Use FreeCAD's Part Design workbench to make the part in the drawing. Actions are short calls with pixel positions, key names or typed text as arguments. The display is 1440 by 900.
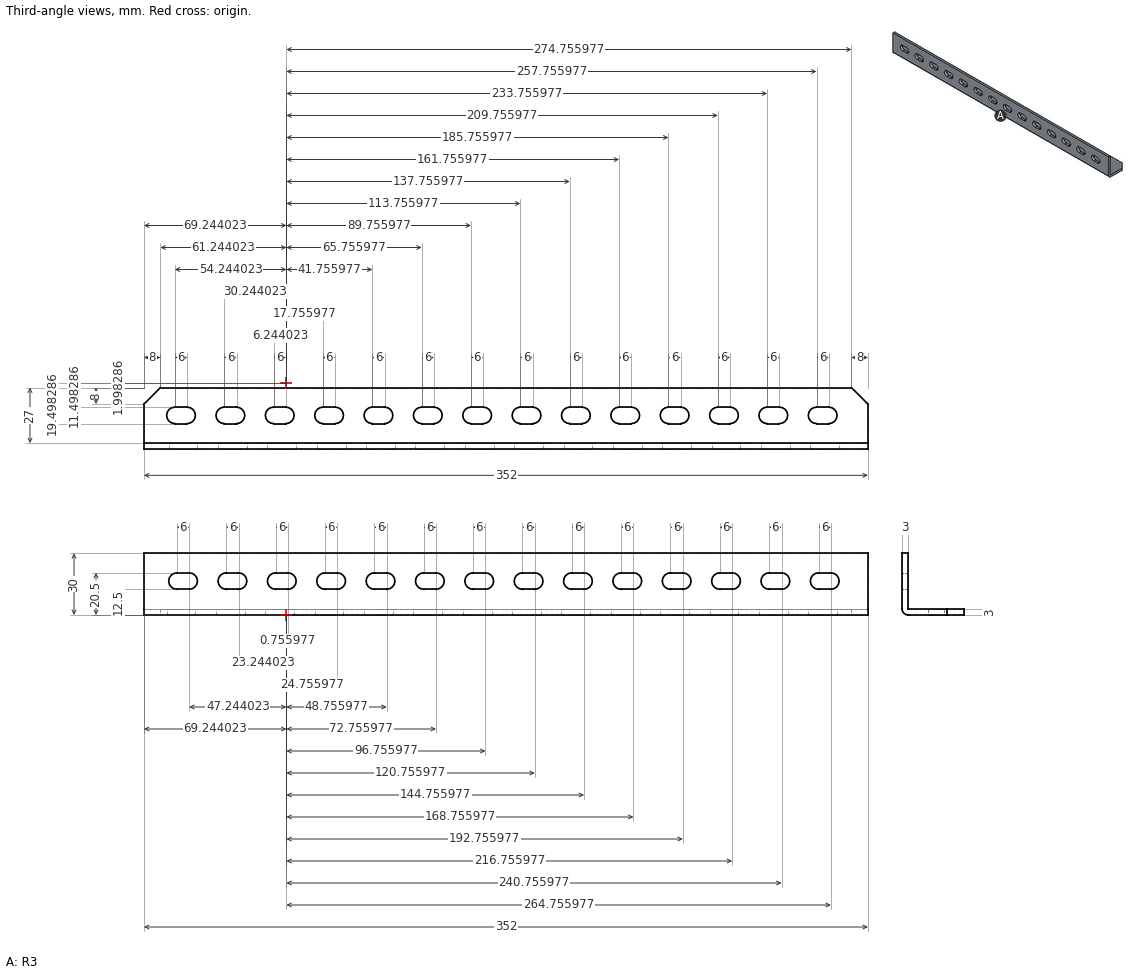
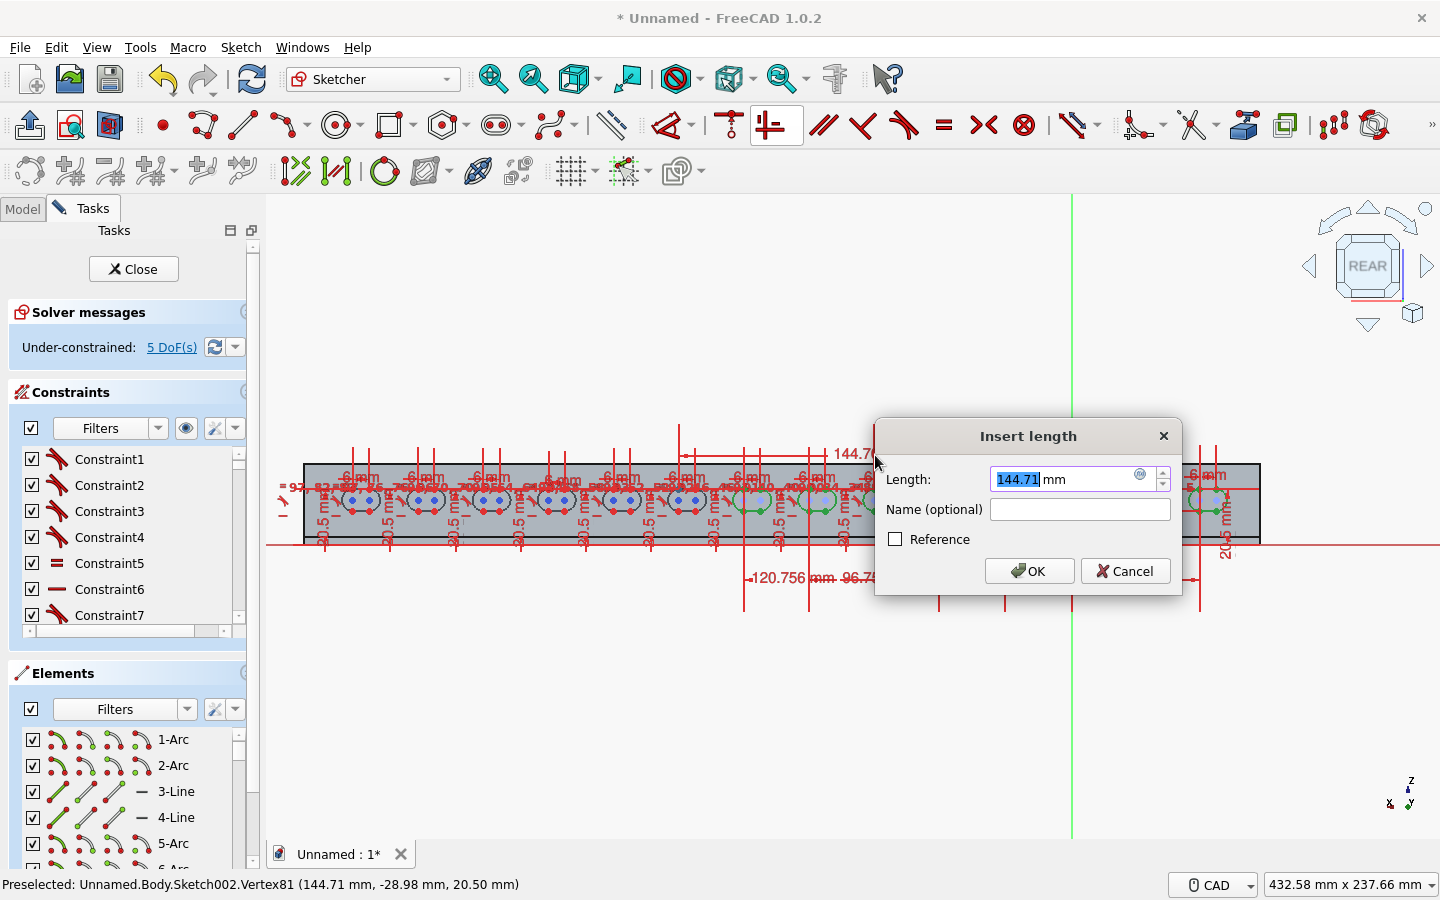
text(144.755977)
key(Return)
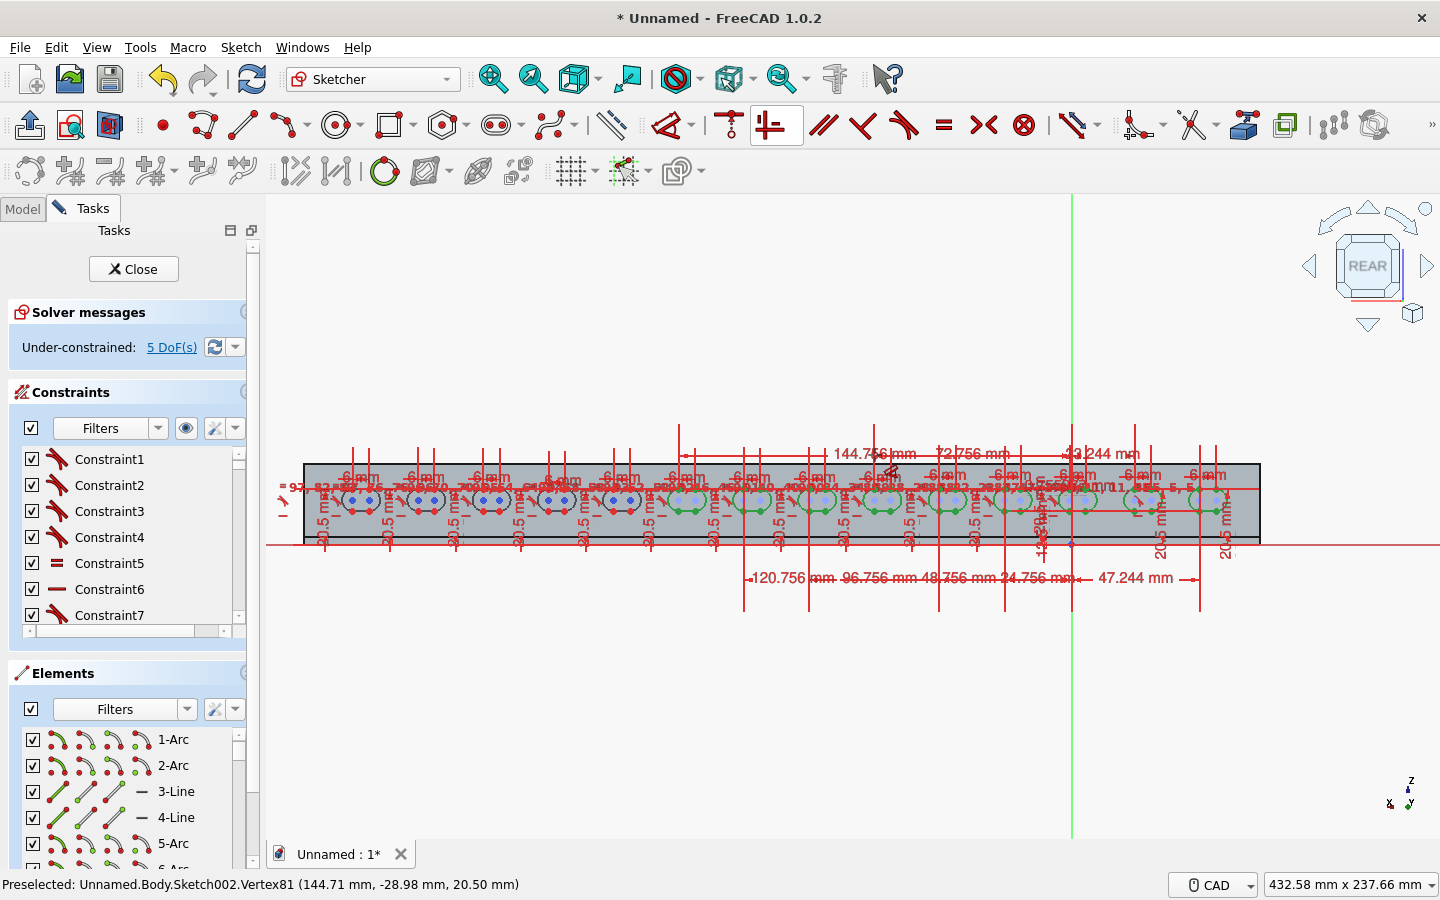
click(614, 489)
click(683, 579)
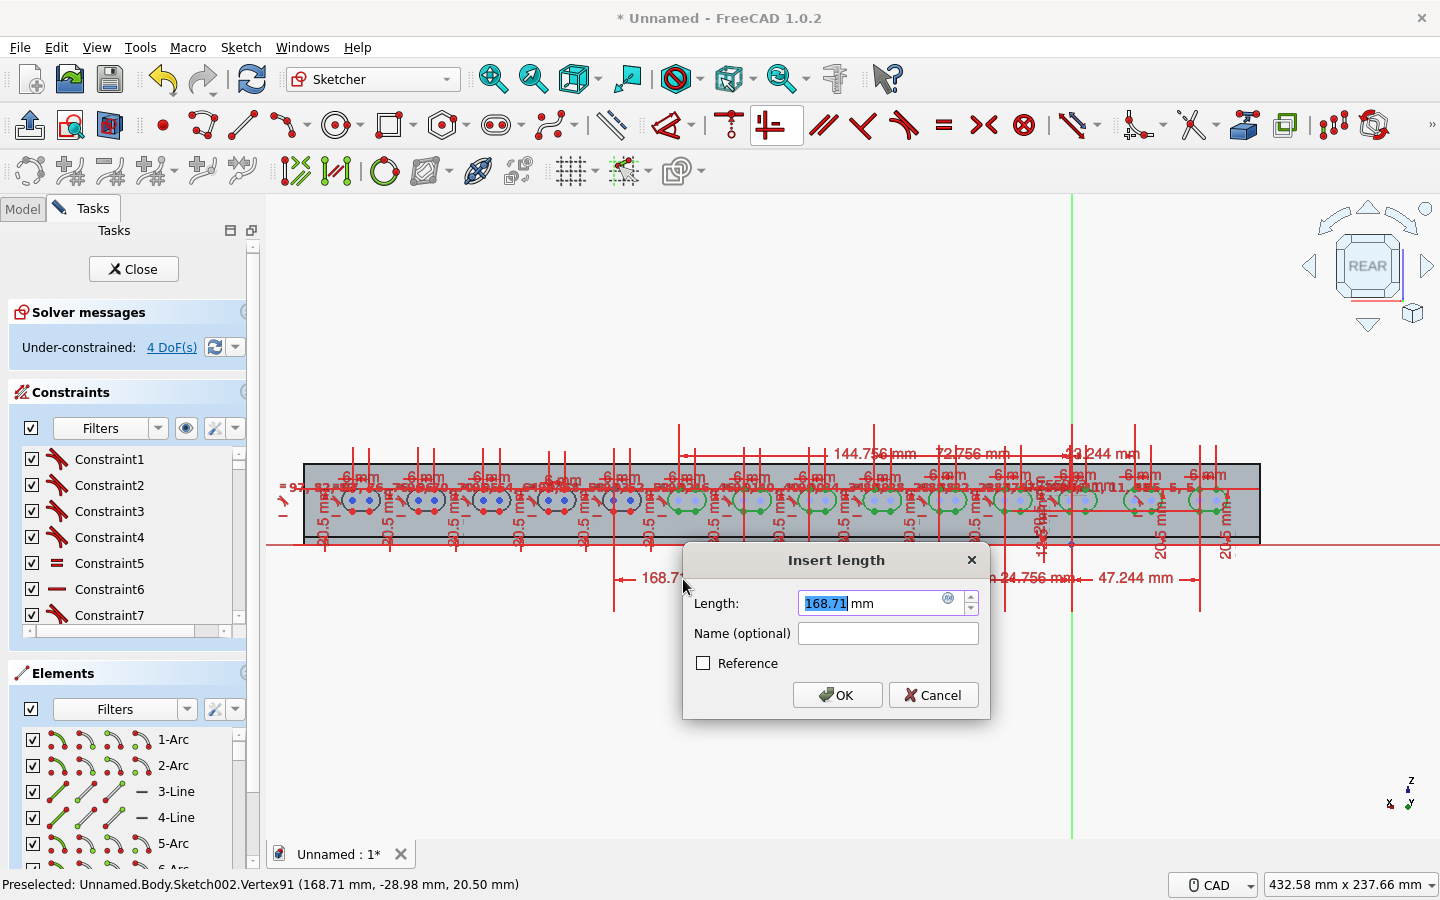
text(168.755977)
key(Return)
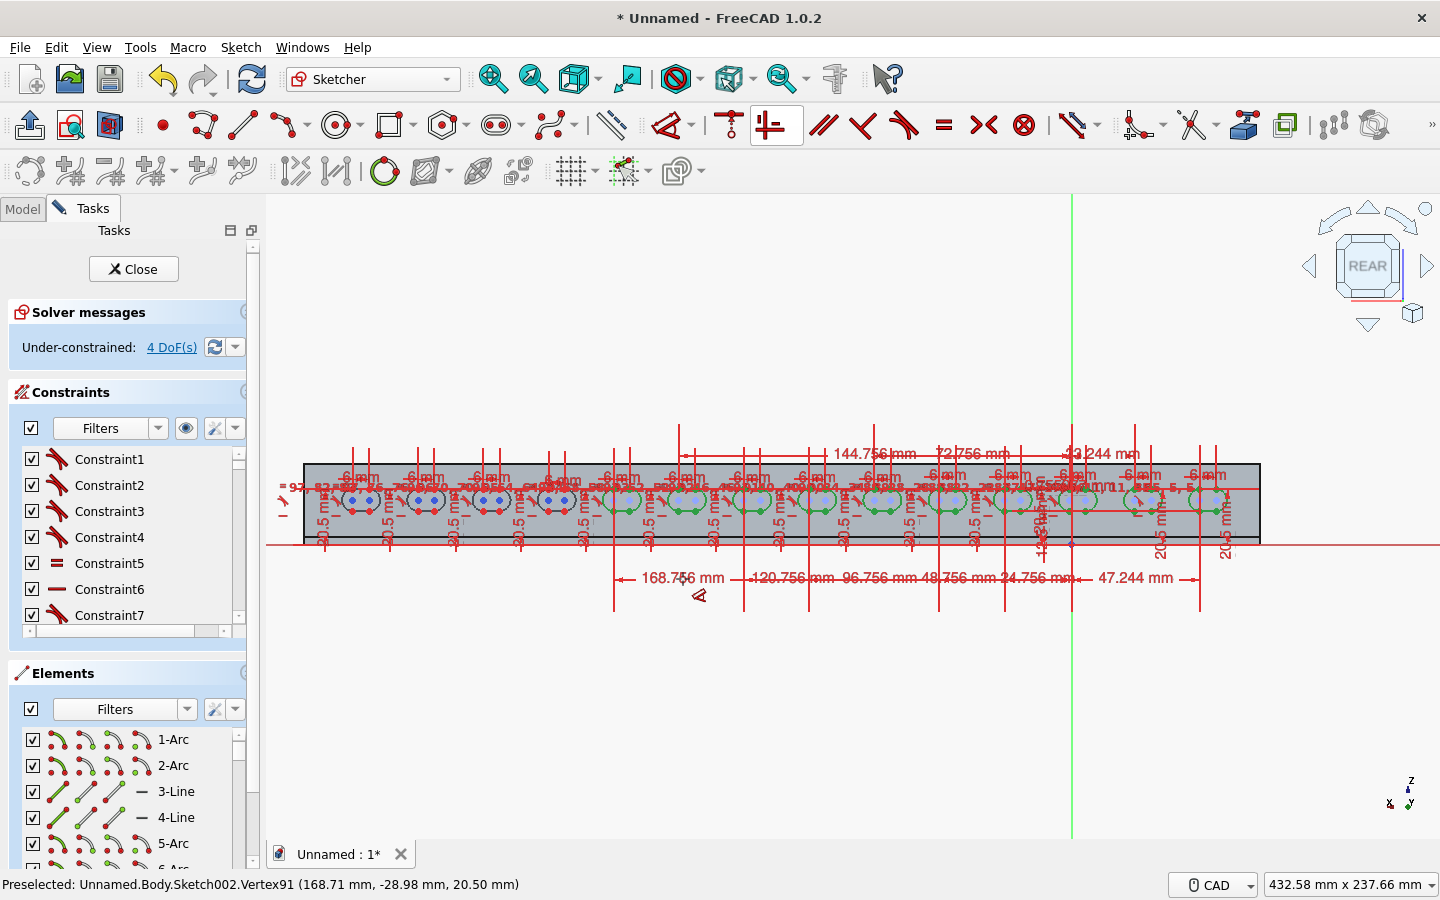
click(549, 489)
click(690, 455)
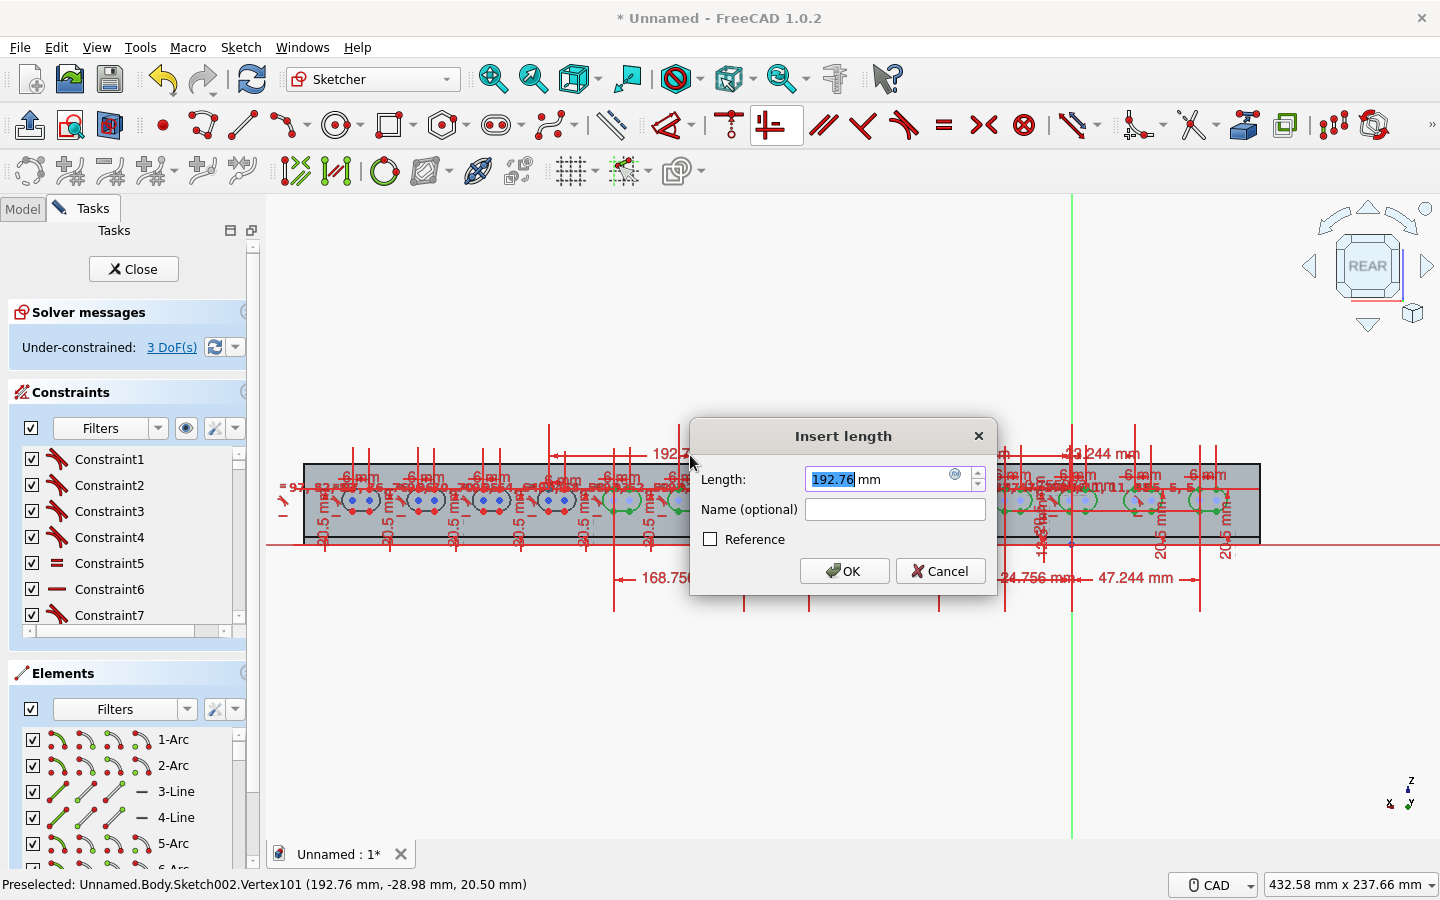
text(192.755977)
key(Return)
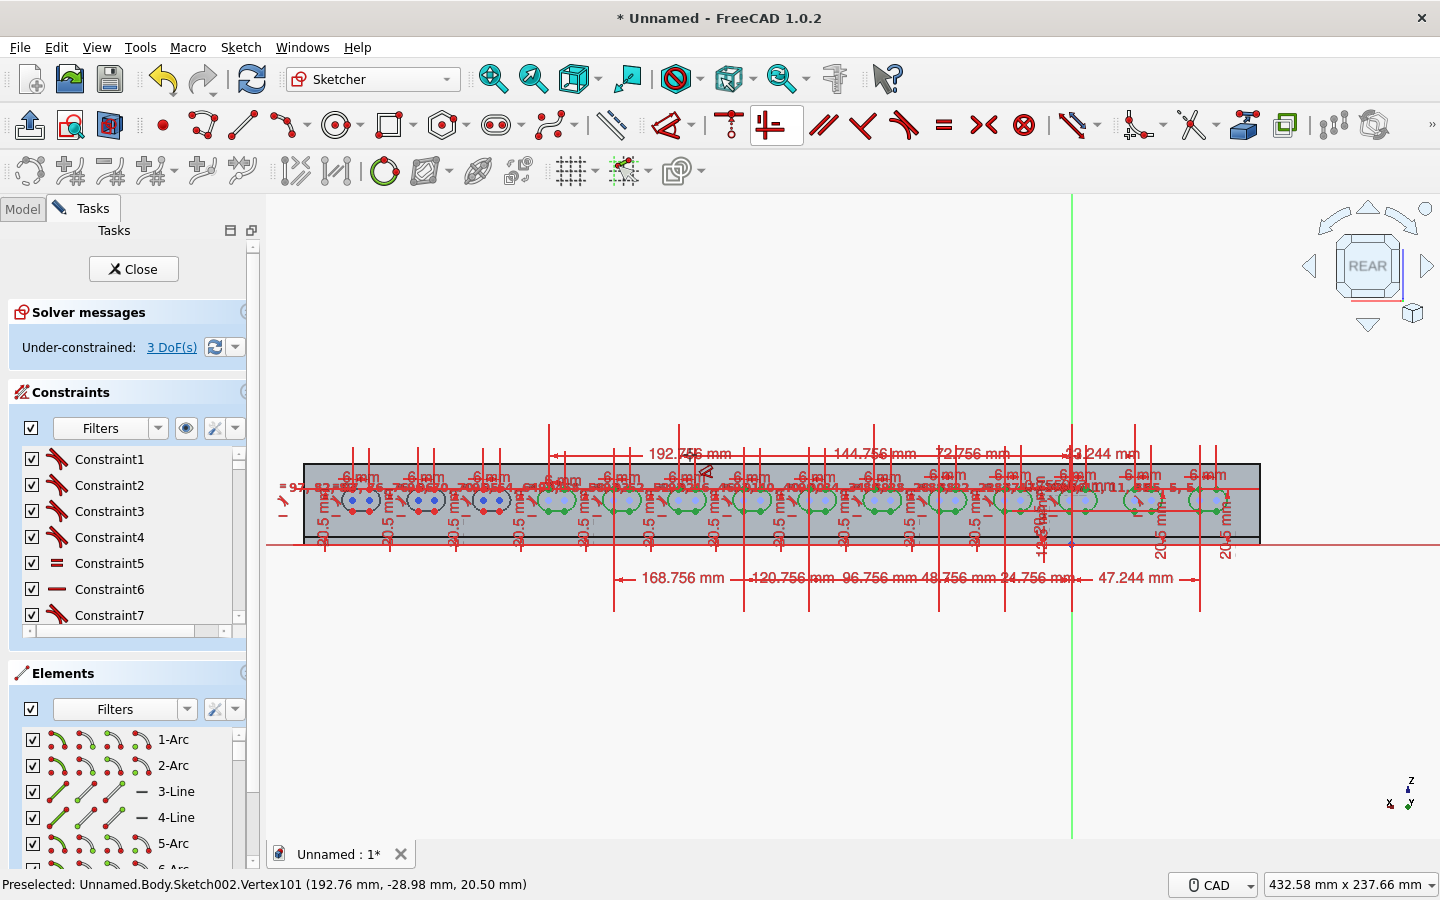
click(483, 489)
click(572, 579)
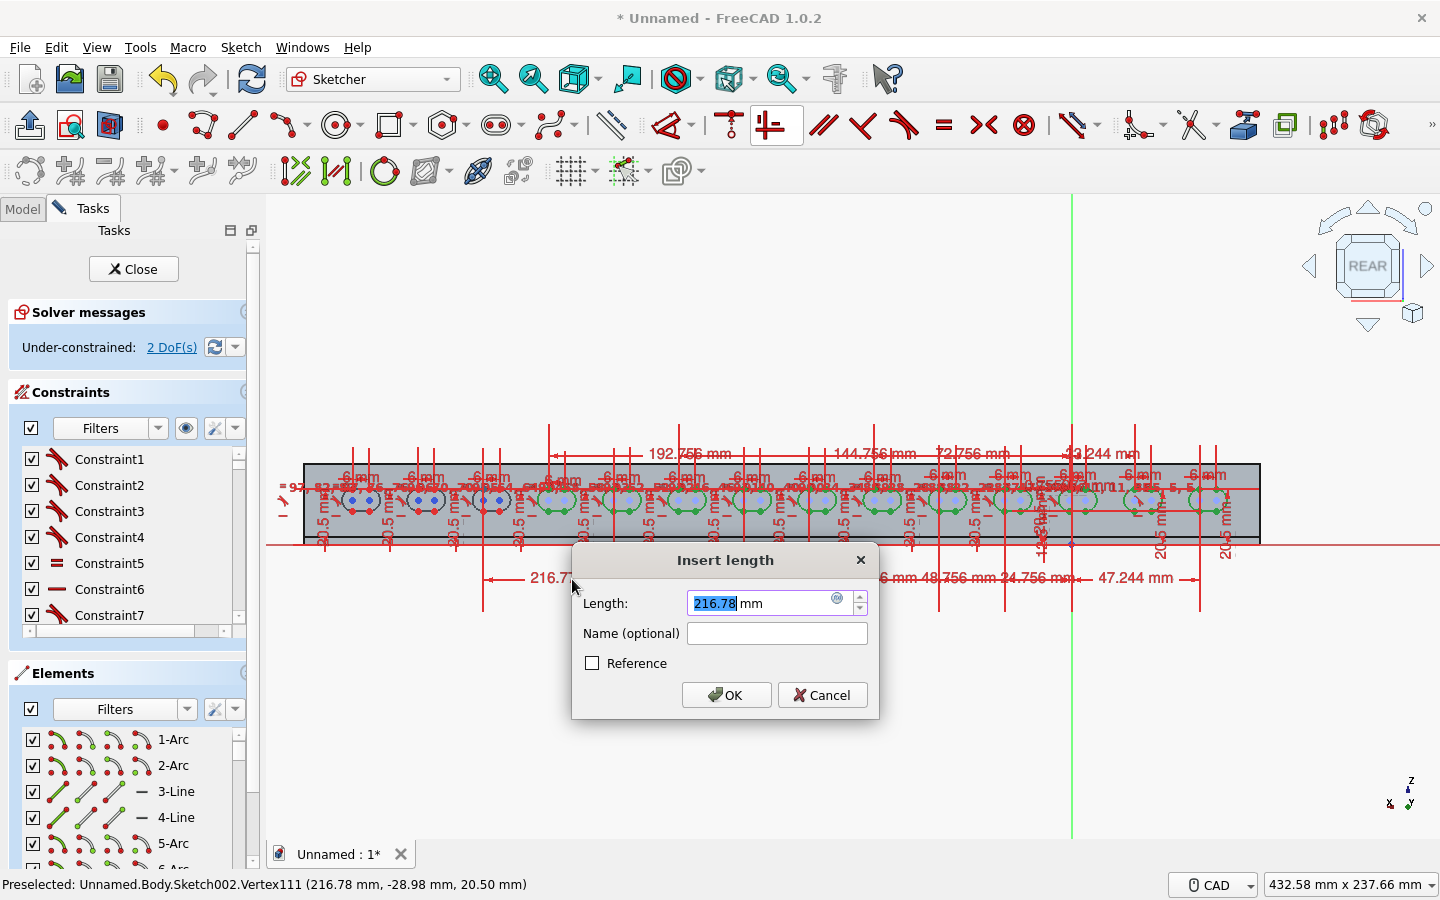
text(216.755977)
key(Return)